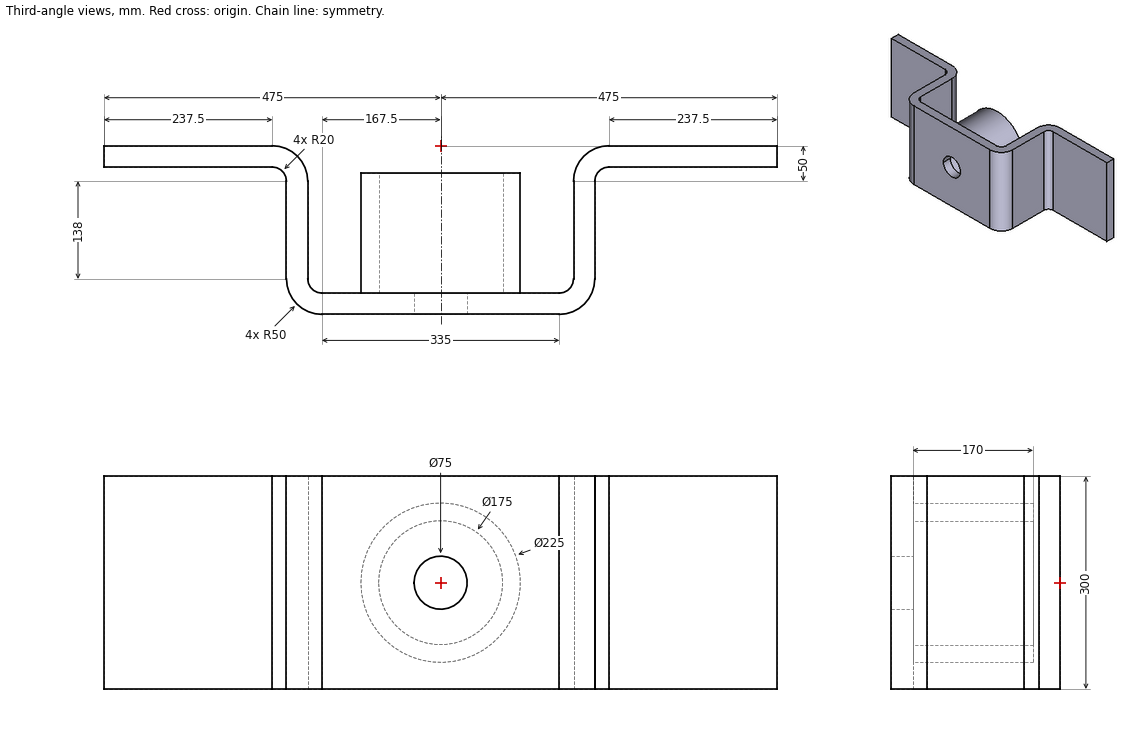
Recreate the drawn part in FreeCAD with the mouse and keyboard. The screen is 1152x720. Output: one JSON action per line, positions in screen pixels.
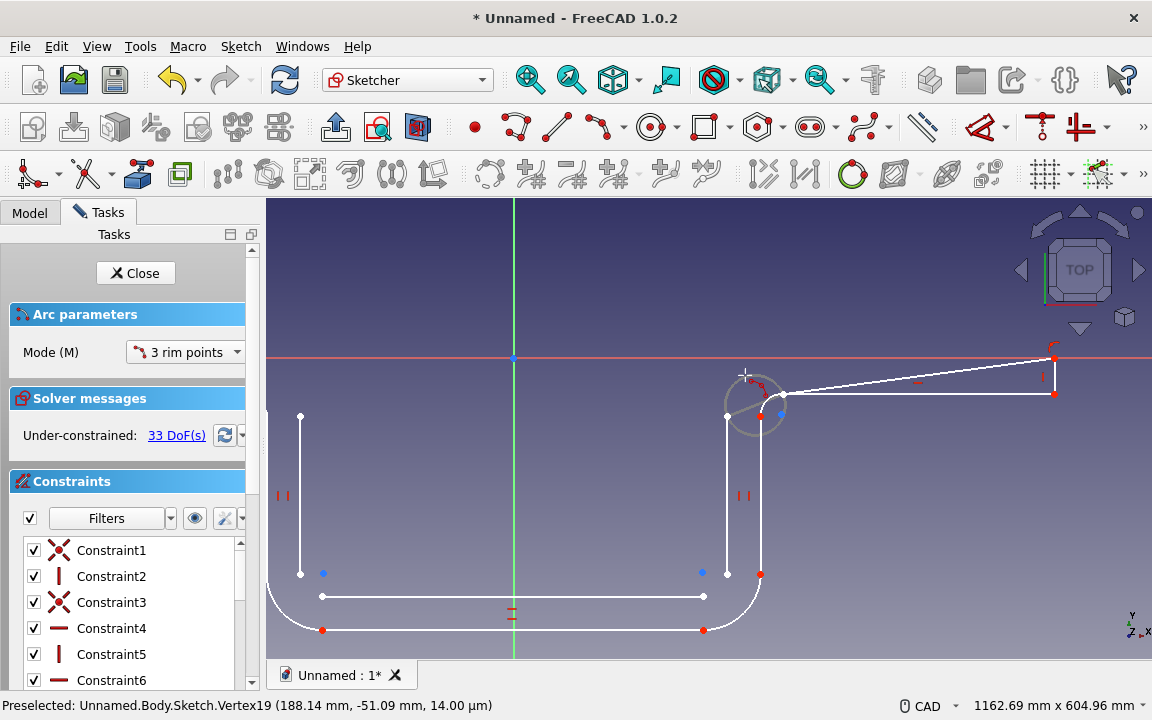
{"action": "left_click", "coordinate": [743, 375]}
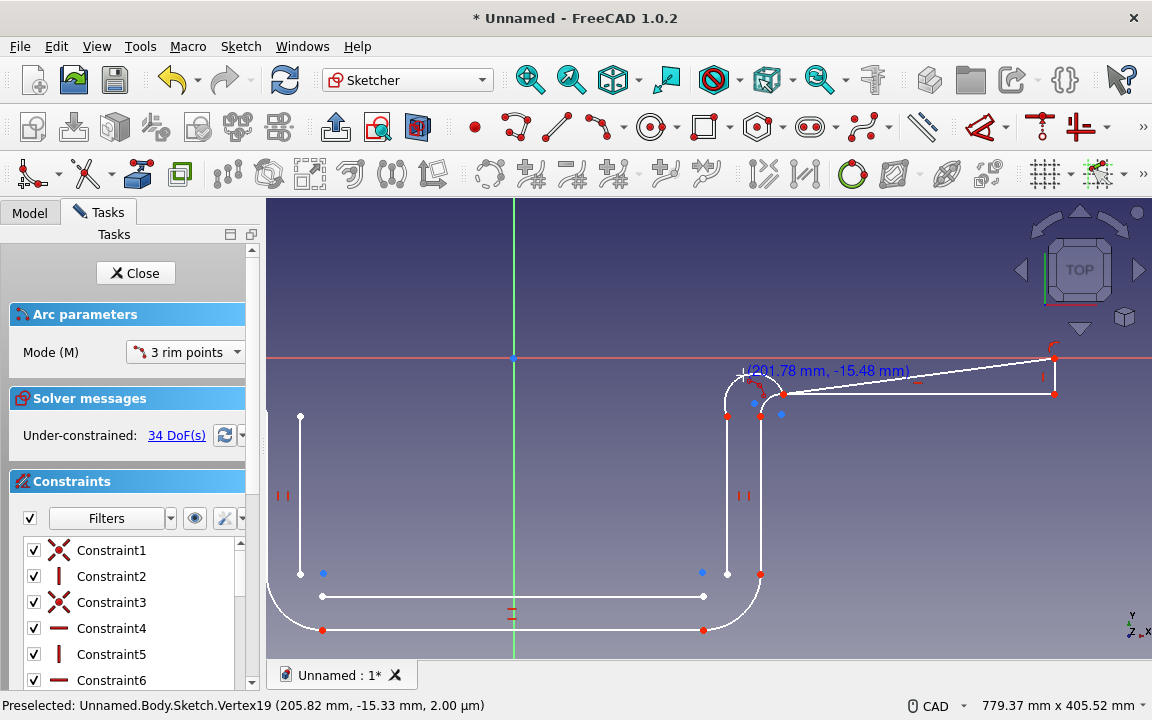
{"action": "left_click", "coordinate": [727, 574]}
{"action": "left_click", "coordinate": [703, 597]}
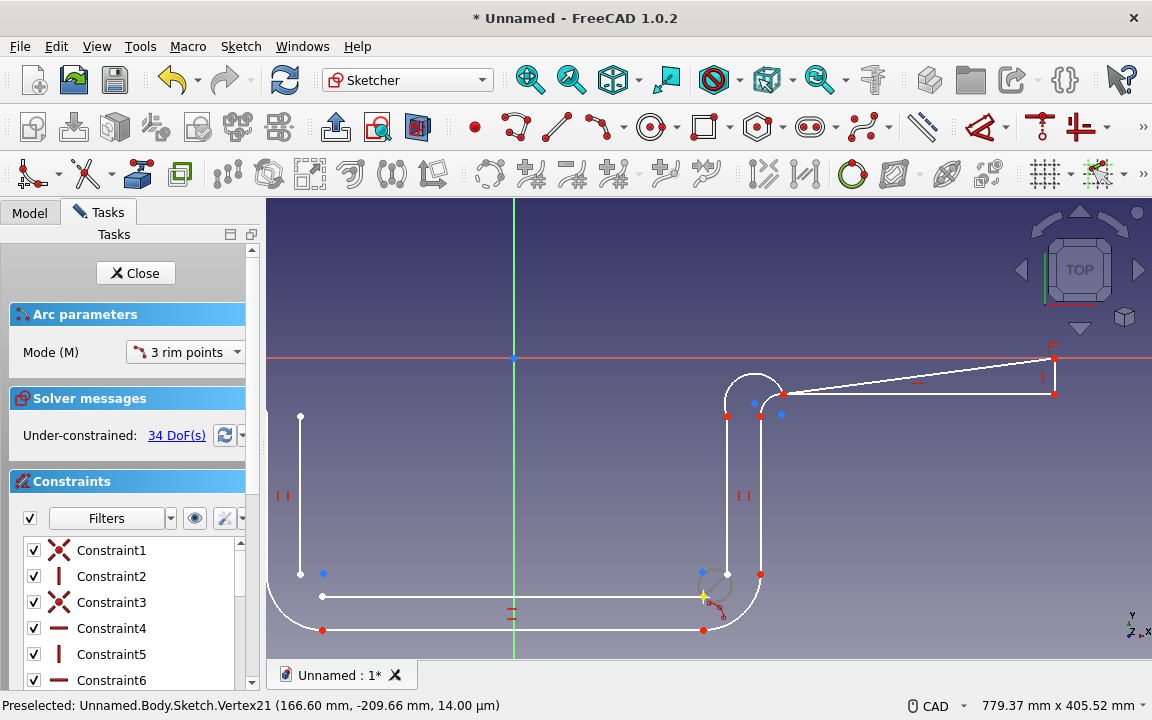
{"action": "scroll", "coordinate": [720, 588], "scroll_direction": "up", "scroll_amount": 5}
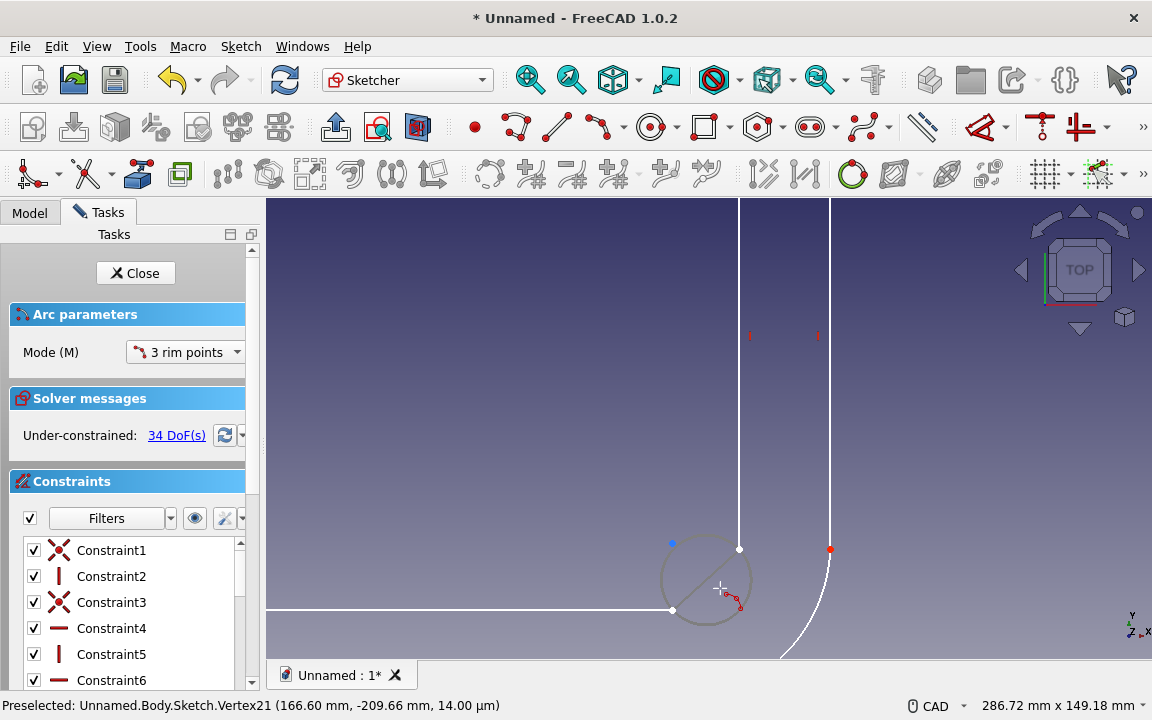
{"action": "left_click", "coordinate": [719, 587]}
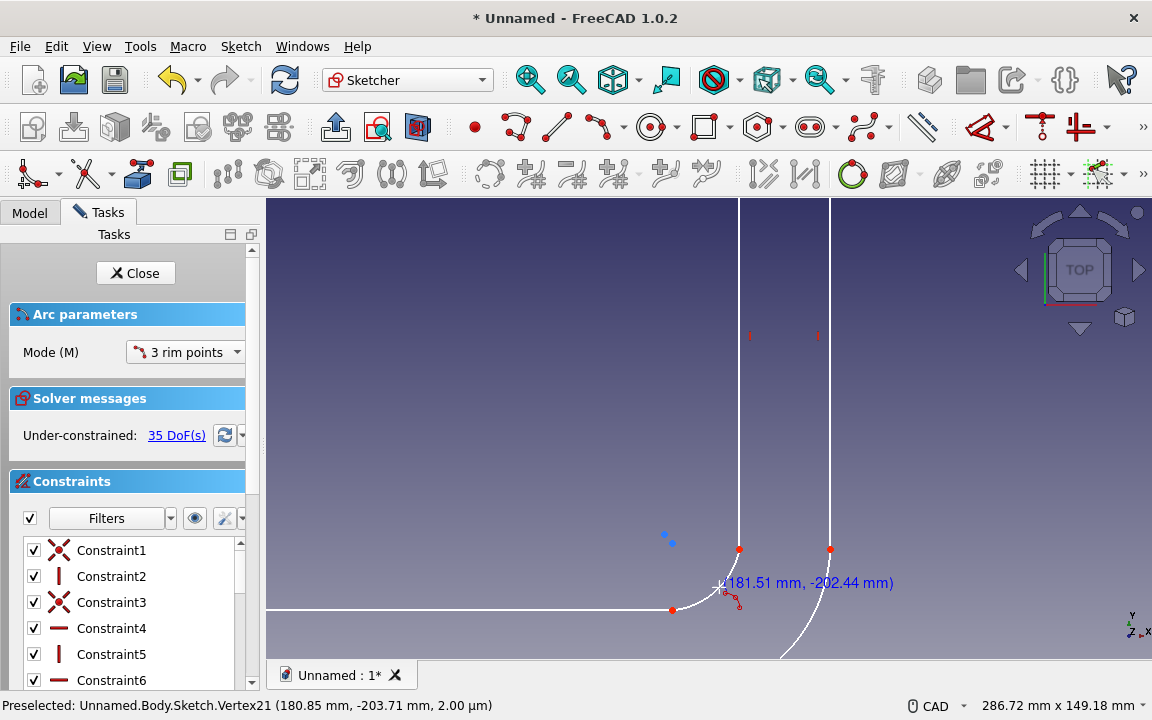
{"action": "scroll", "coordinate": [736, 448], "scroll_direction": "down", "scroll_amount": 9}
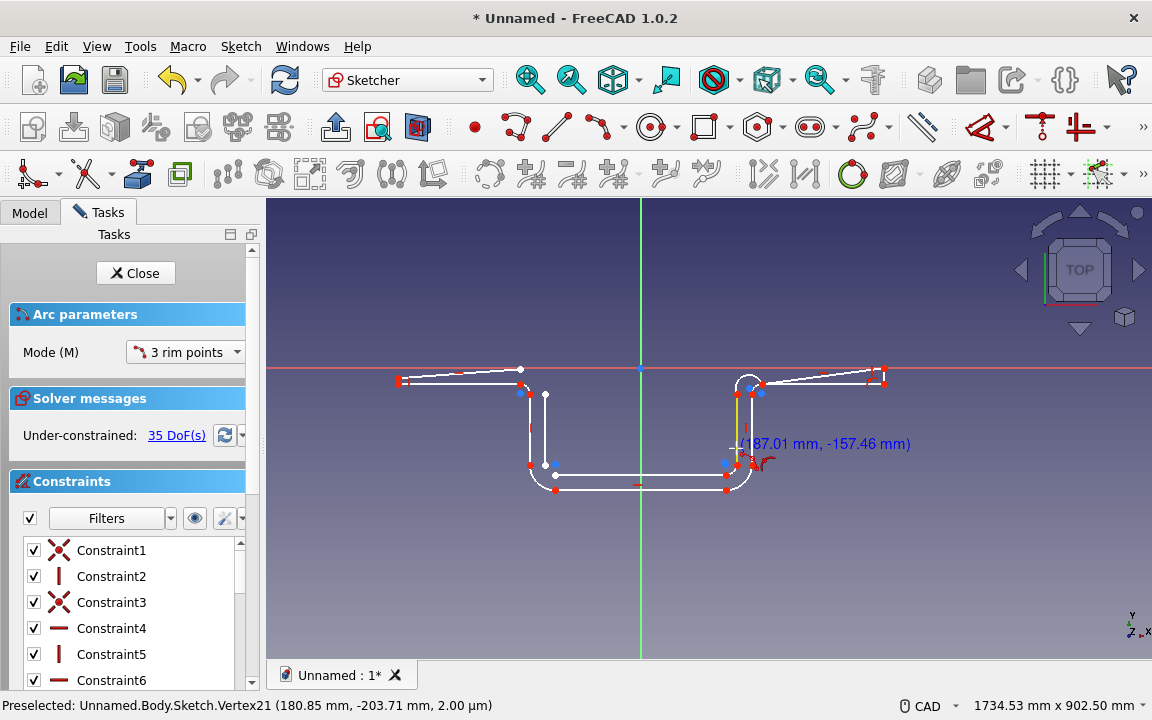
{"action": "scroll", "coordinate": [555, 474], "scroll_direction": "up", "scroll_amount": 3}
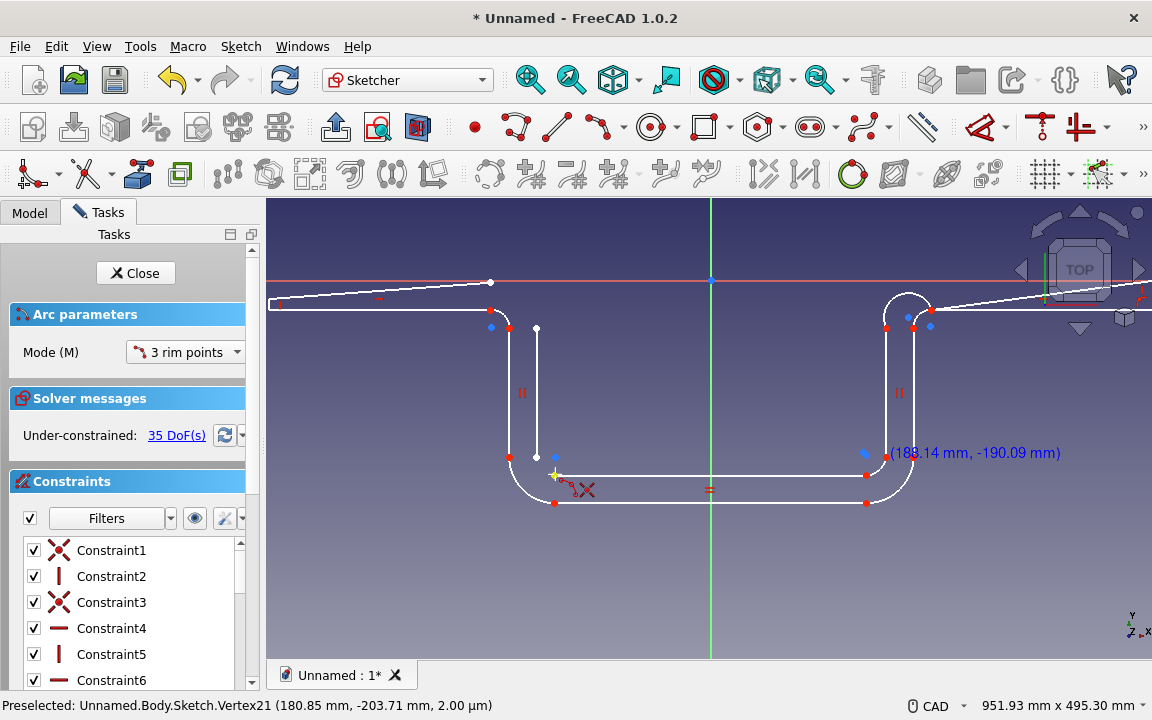
{"action": "left_click", "coordinate": [555, 476]}
{"action": "left_click", "coordinate": [537, 458]}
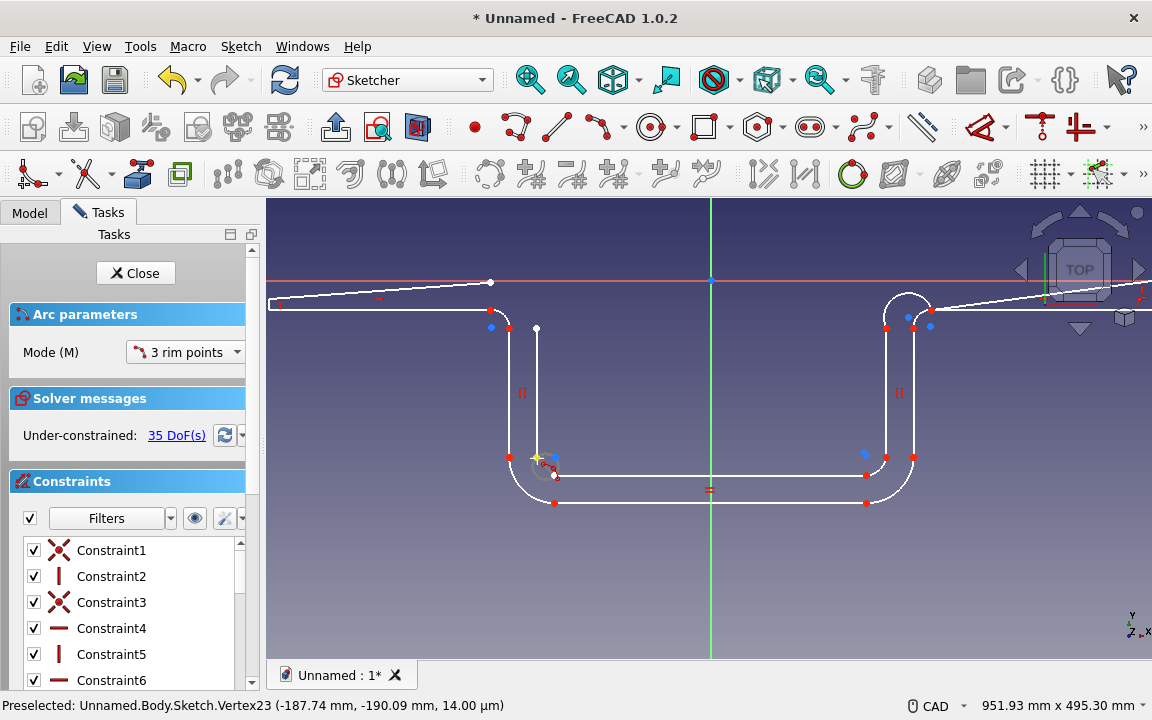
{"action": "scroll", "coordinate": [542, 469], "scroll_direction": "up", "scroll_amount": 6}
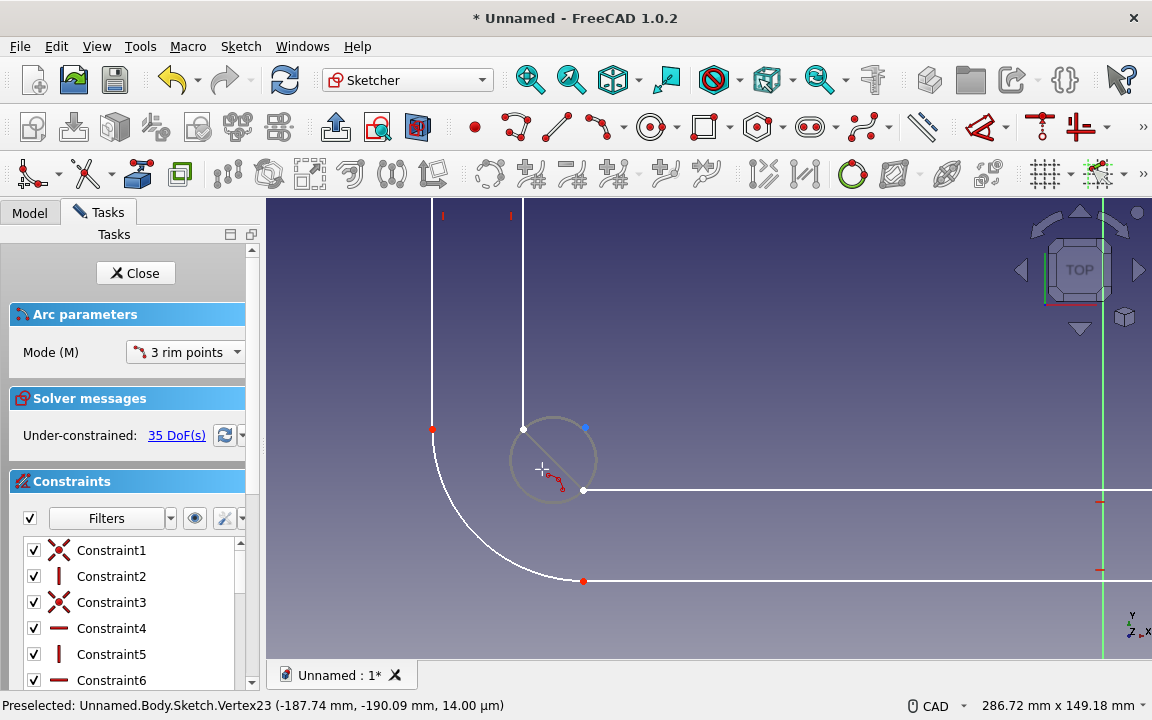
{"action": "left_click", "coordinate": [542, 467]}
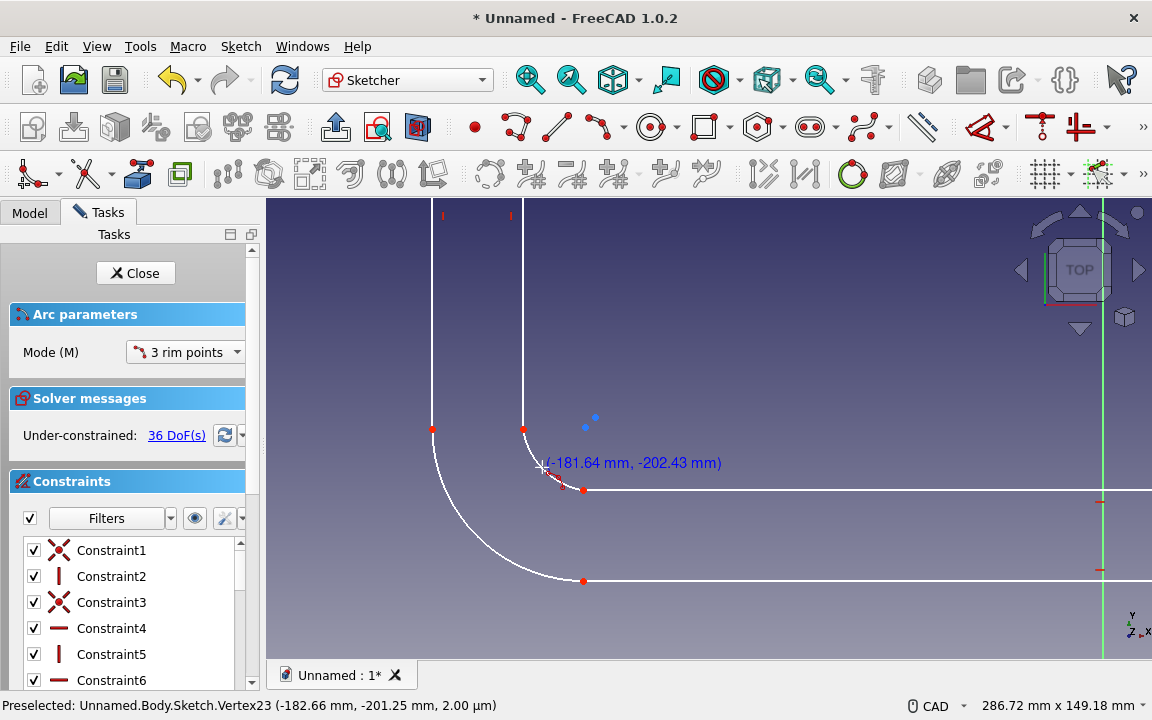
{"action": "scroll", "coordinate": [549, 472], "scroll_direction": "down", "scroll_amount": 9}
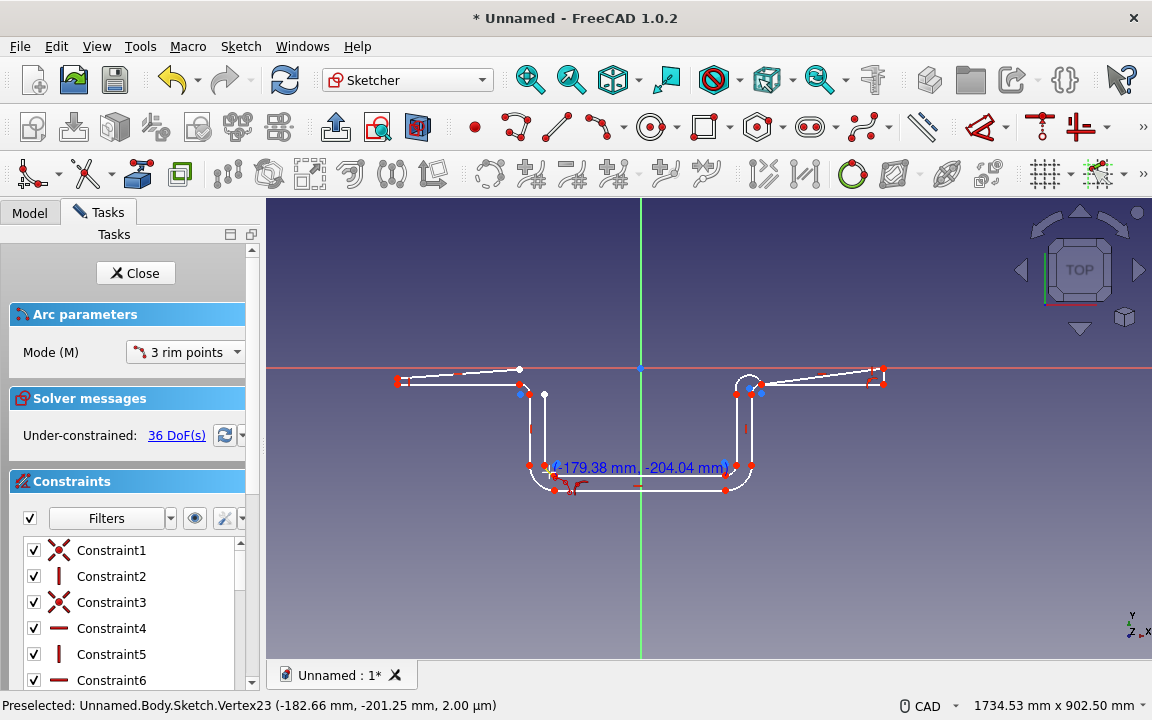
{"action": "left_click", "coordinate": [545, 395]}
{"action": "left_click", "coordinate": [520, 370]}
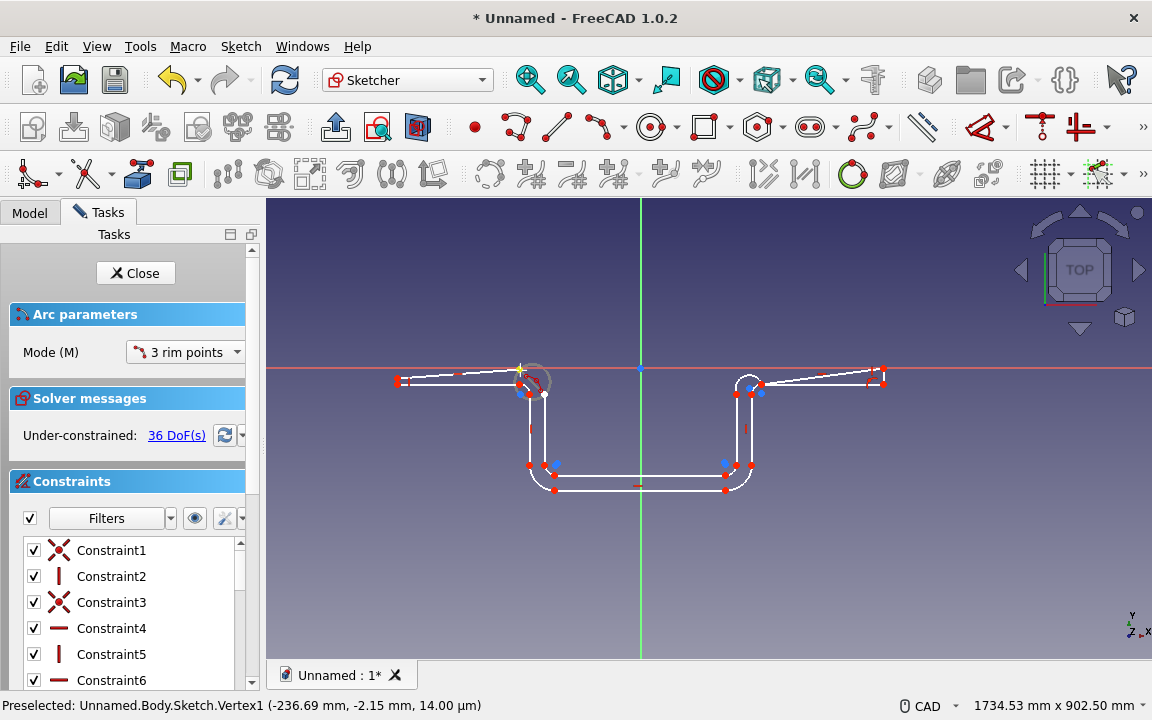
{"action": "scroll", "coordinate": [538, 376], "scroll_direction": "up", "scroll_amount": 4}